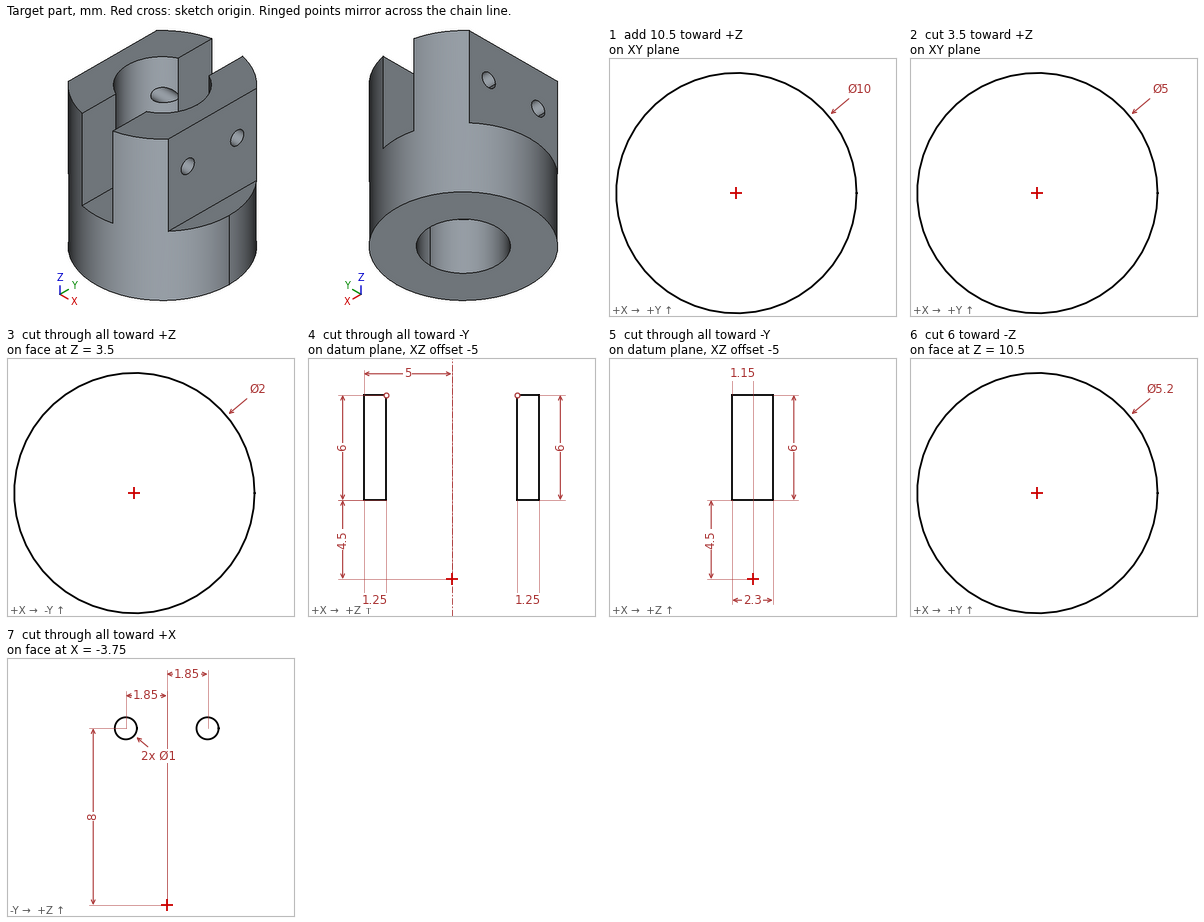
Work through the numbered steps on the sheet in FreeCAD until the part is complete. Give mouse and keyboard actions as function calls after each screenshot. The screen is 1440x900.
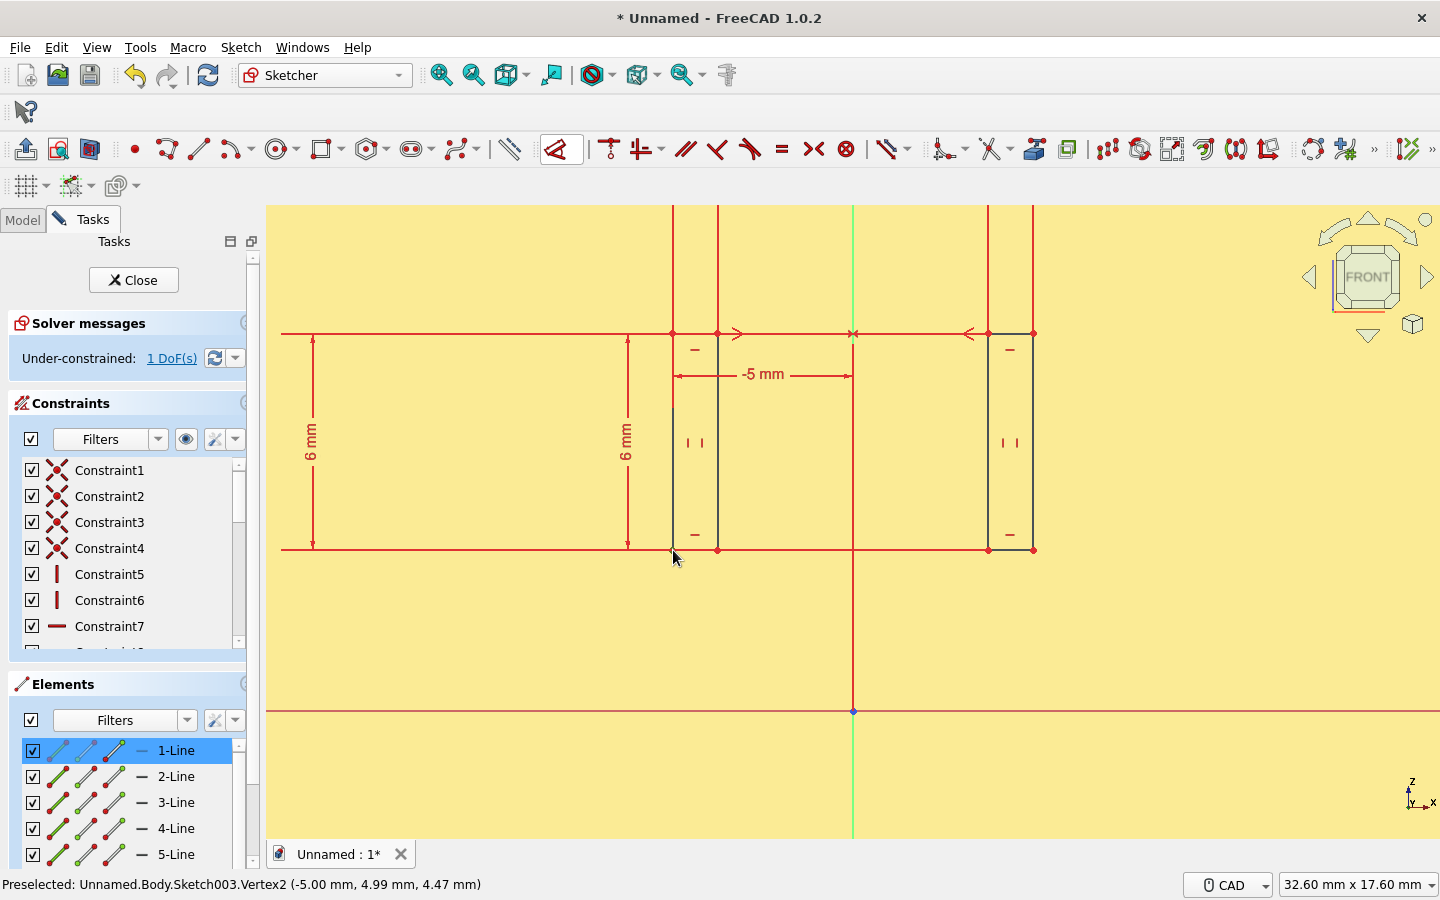
key(i)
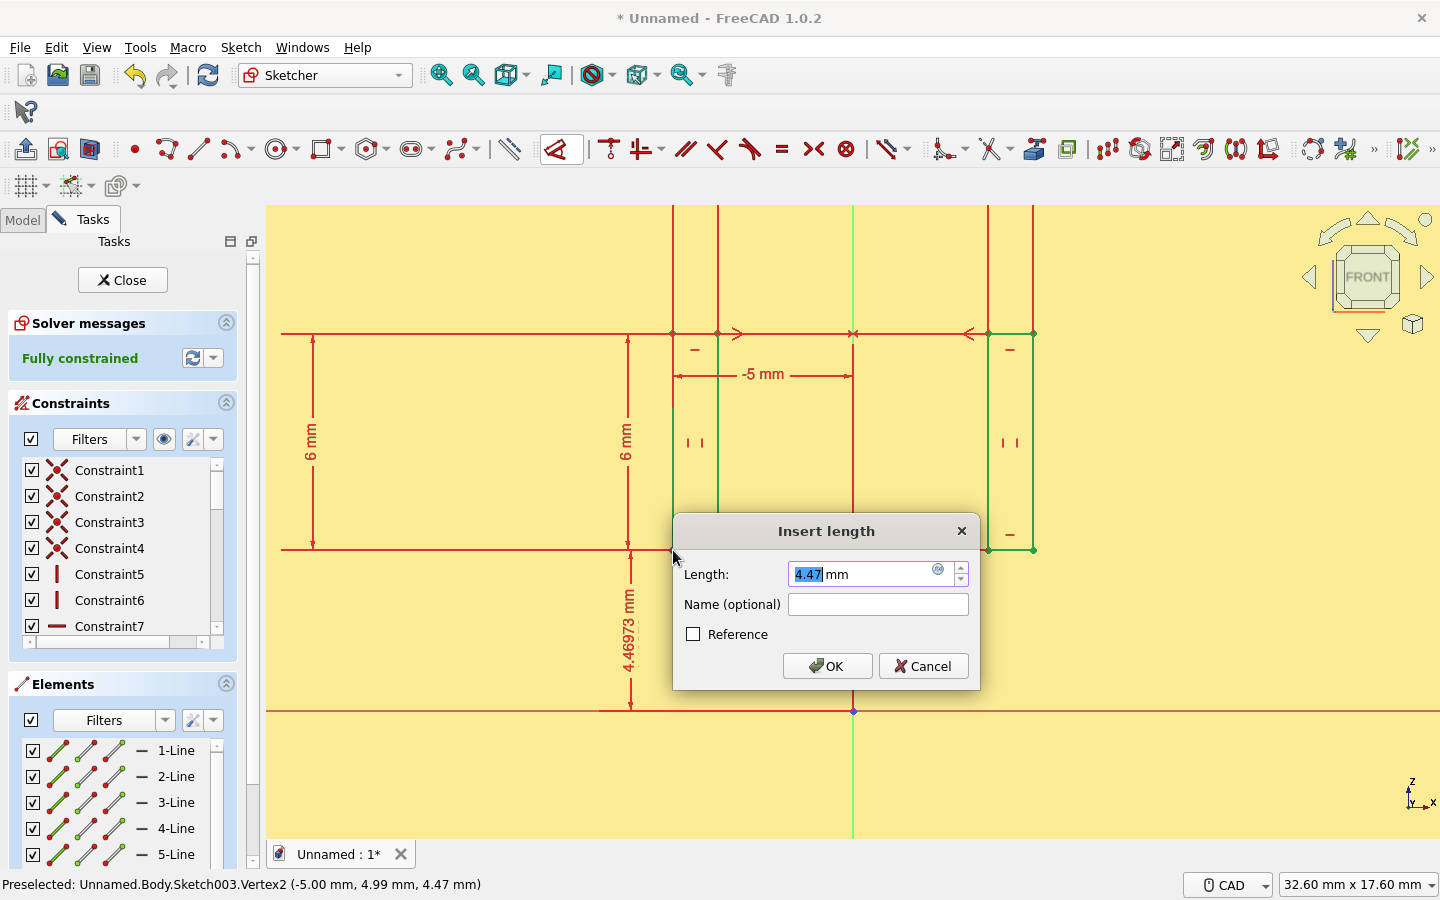
text(4.5)
key(Return)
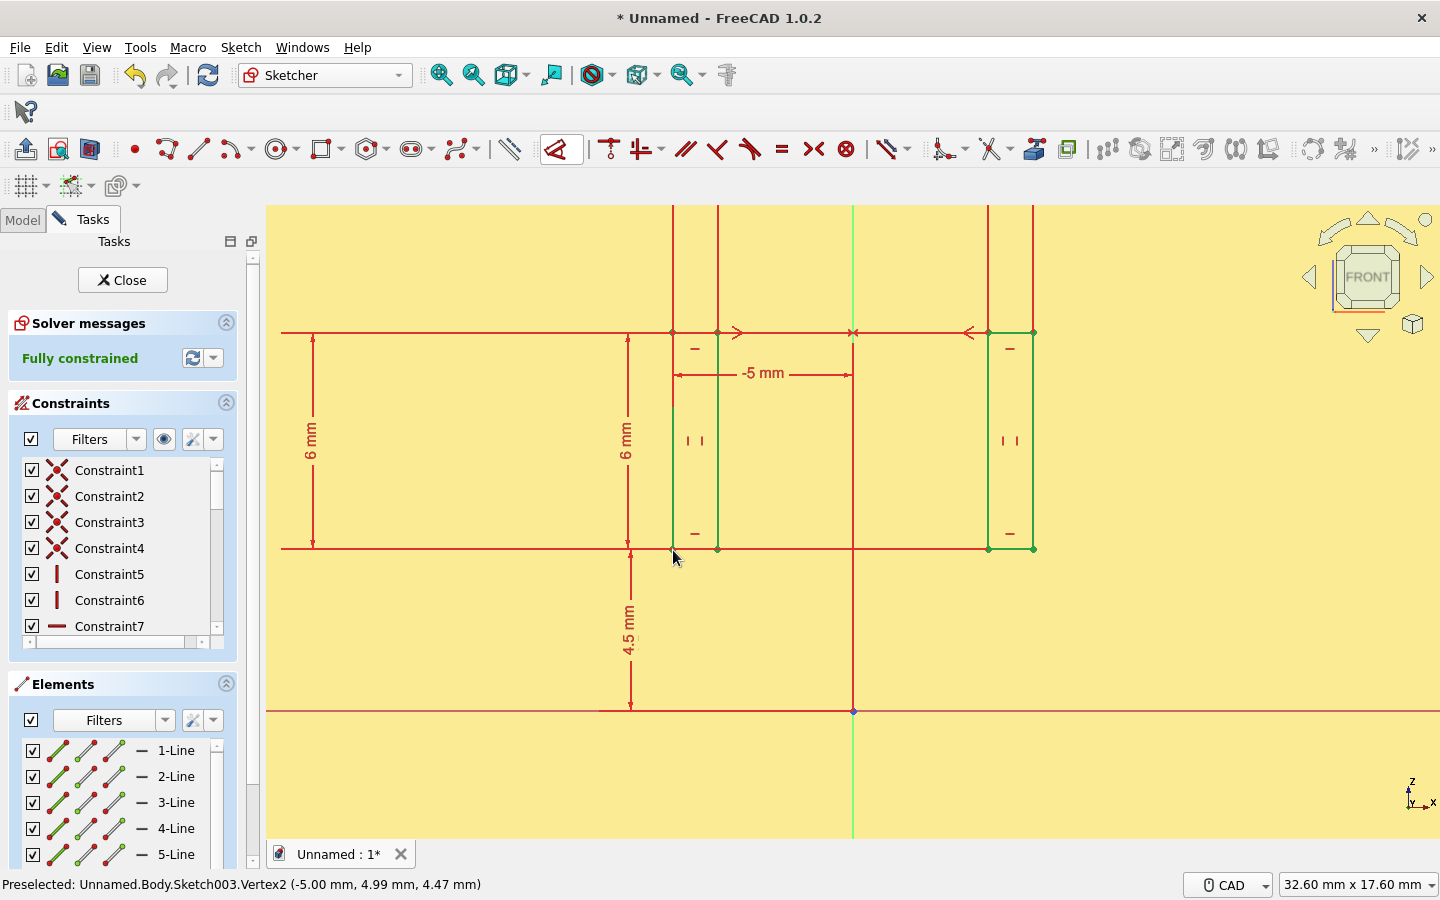
click(123, 280)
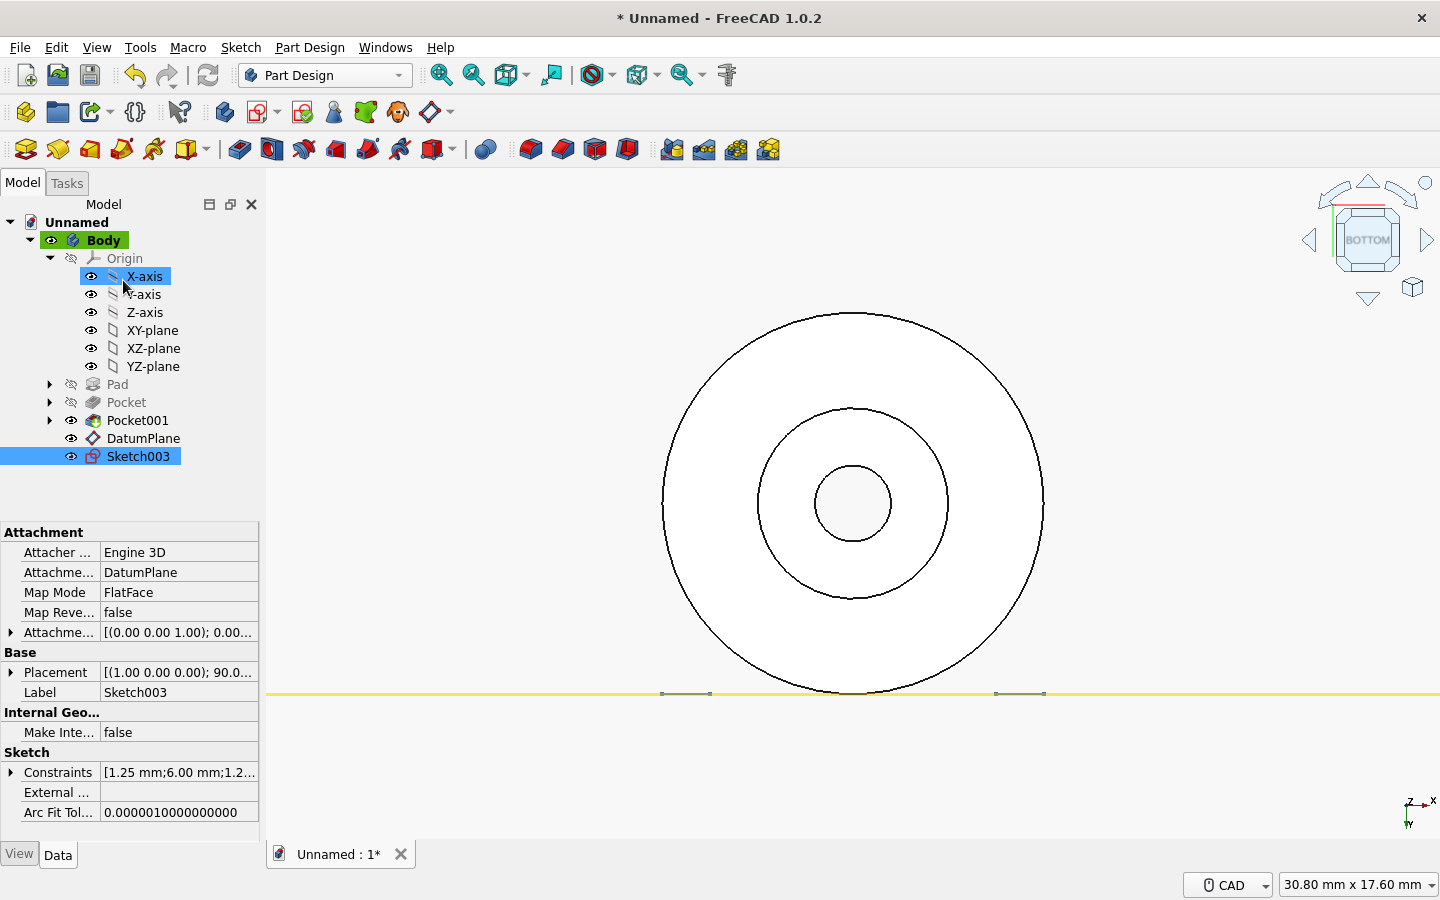
click(240, 150)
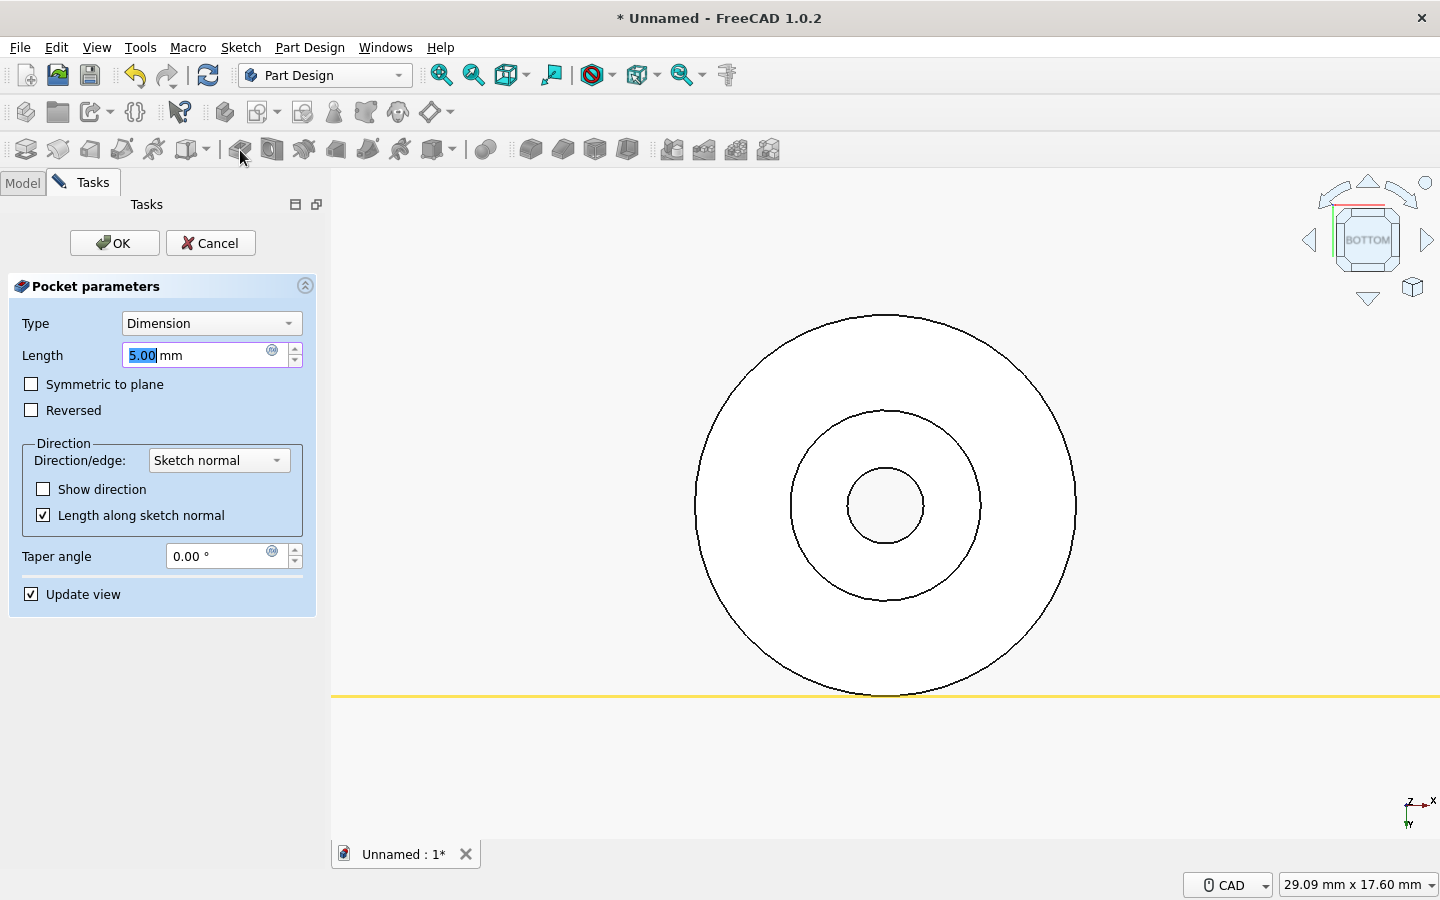
click(212, 324)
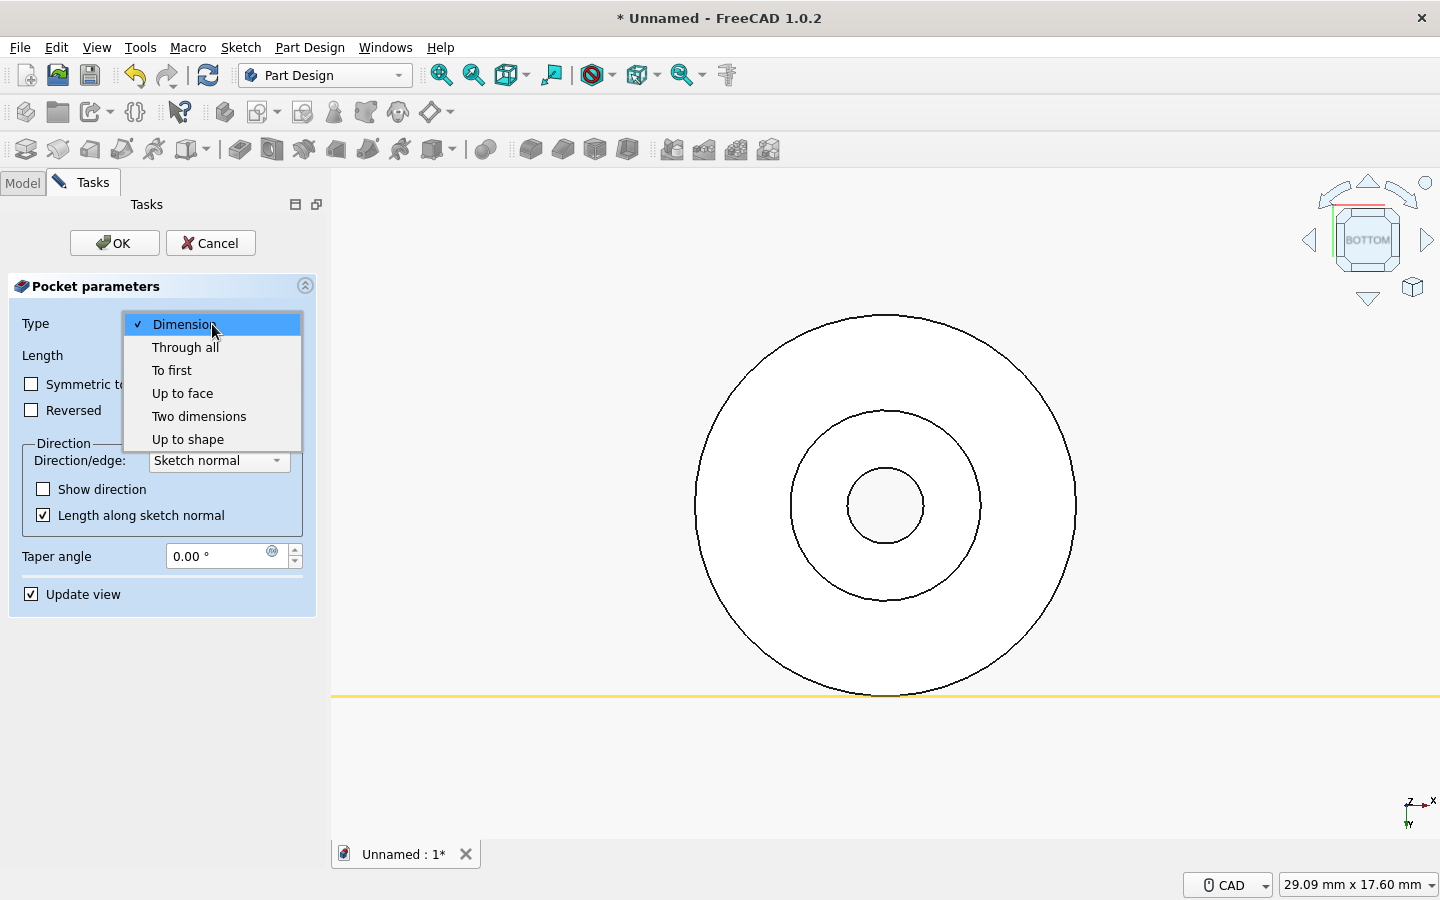
click(212, 348)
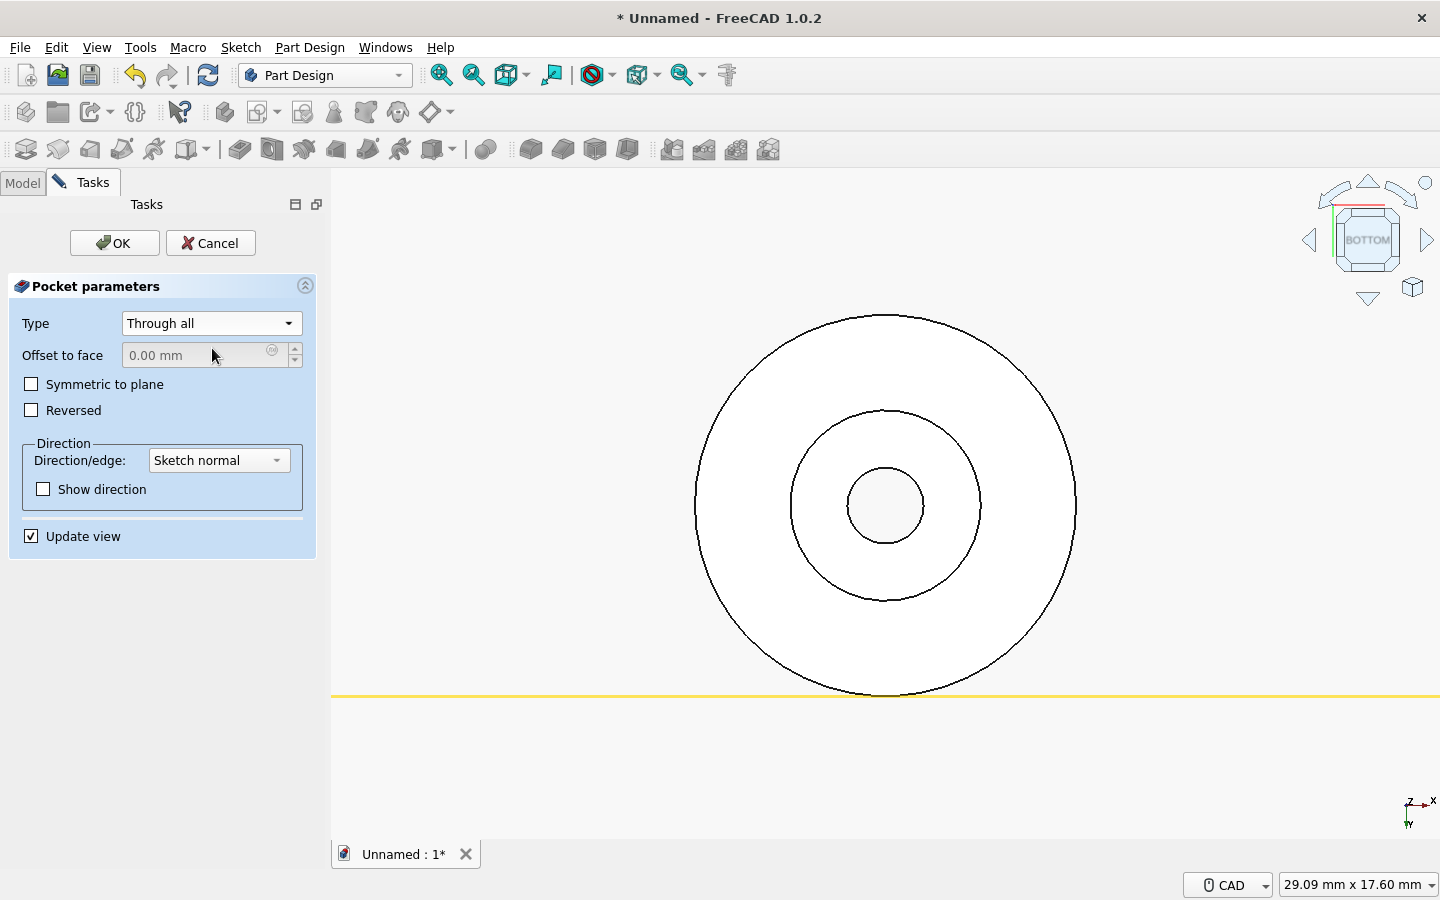
click(30, 410)